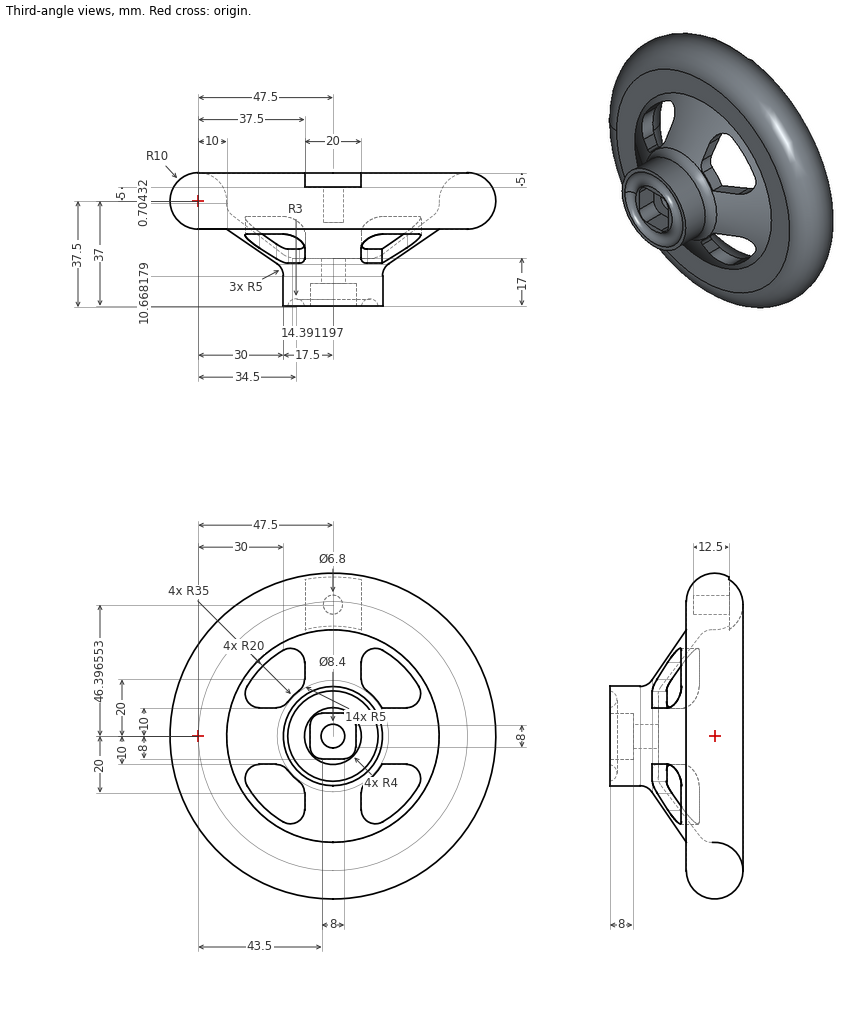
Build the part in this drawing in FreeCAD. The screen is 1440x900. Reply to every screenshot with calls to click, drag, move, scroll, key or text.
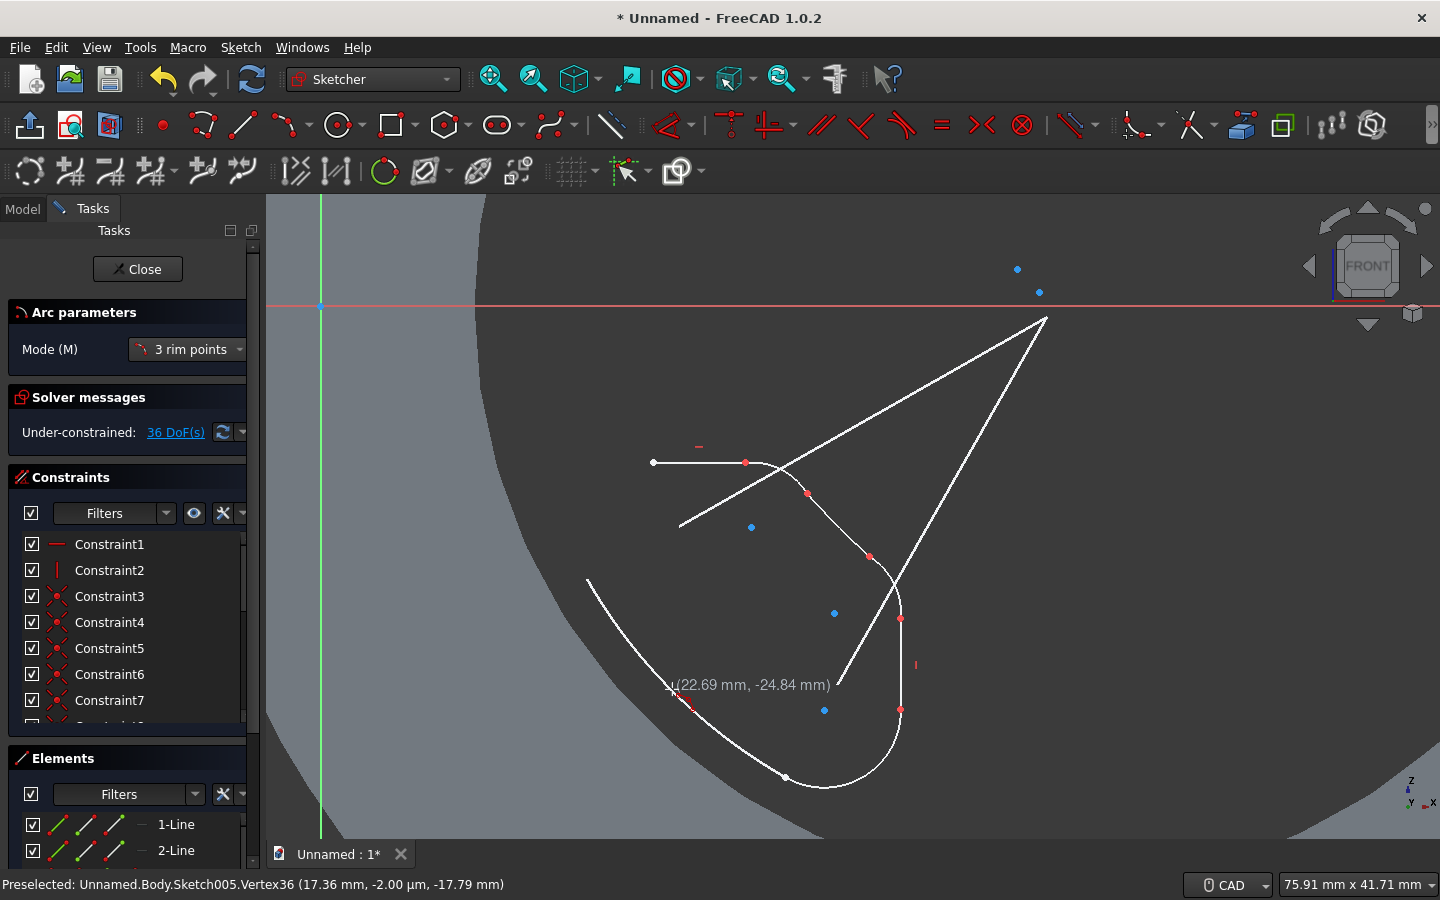
click(673, 689)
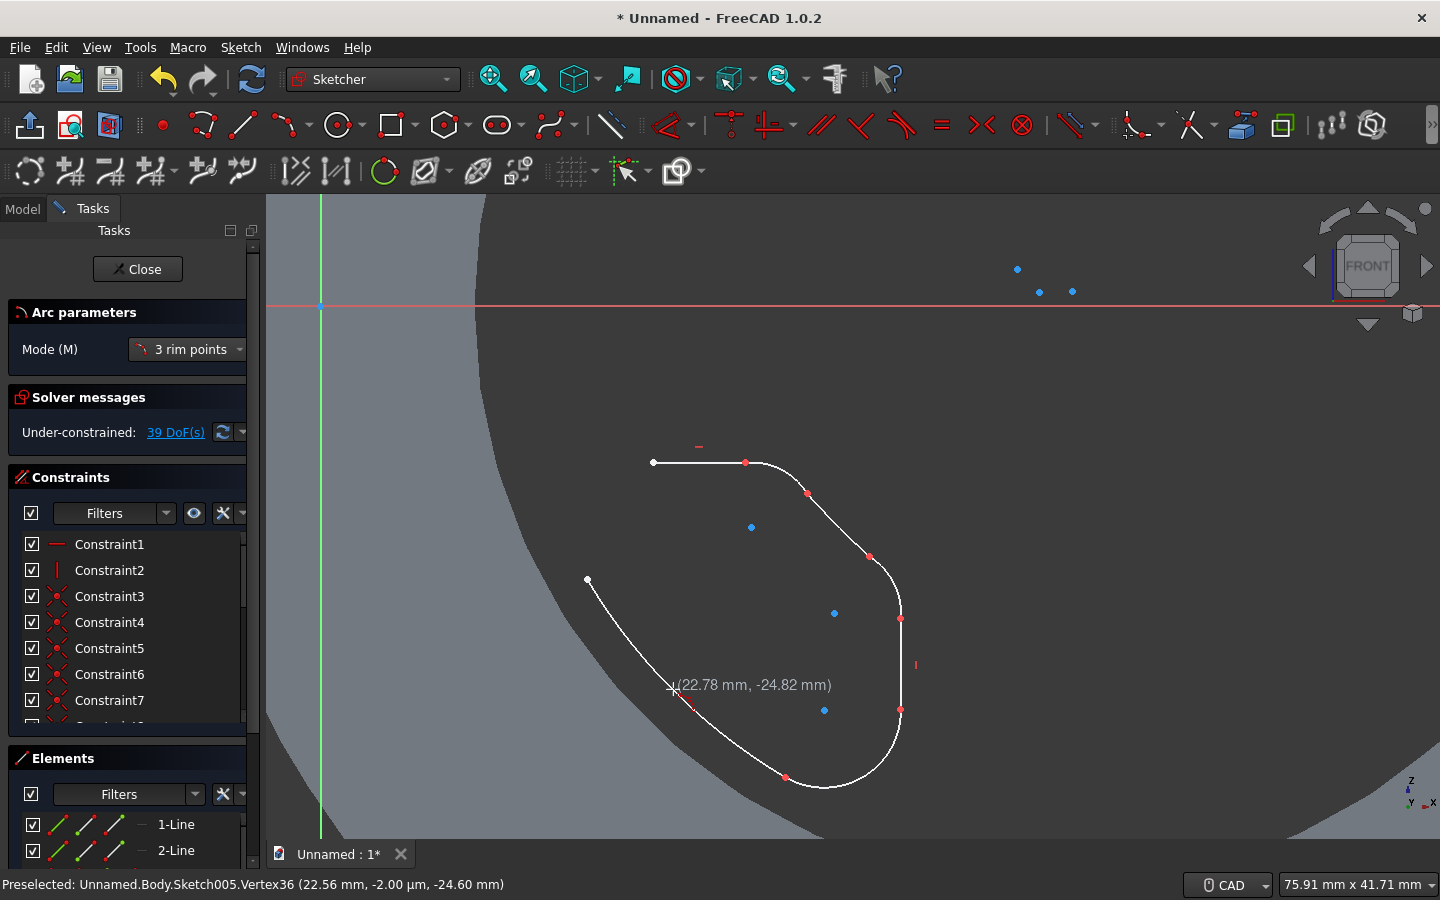
click(587, 579)
click(654, 463)
click(587, 499)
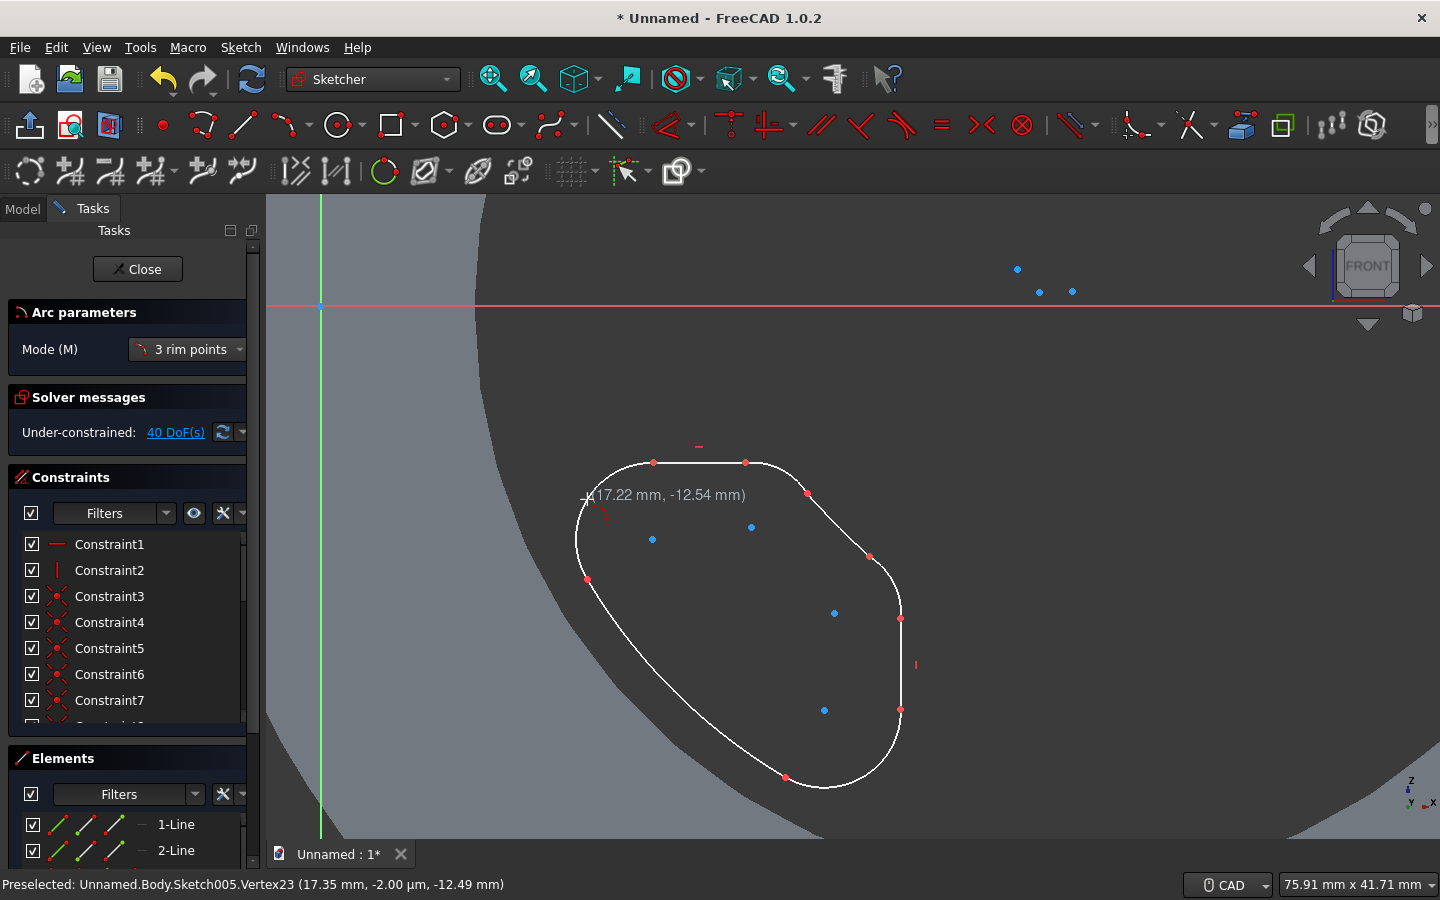
click(244, 126)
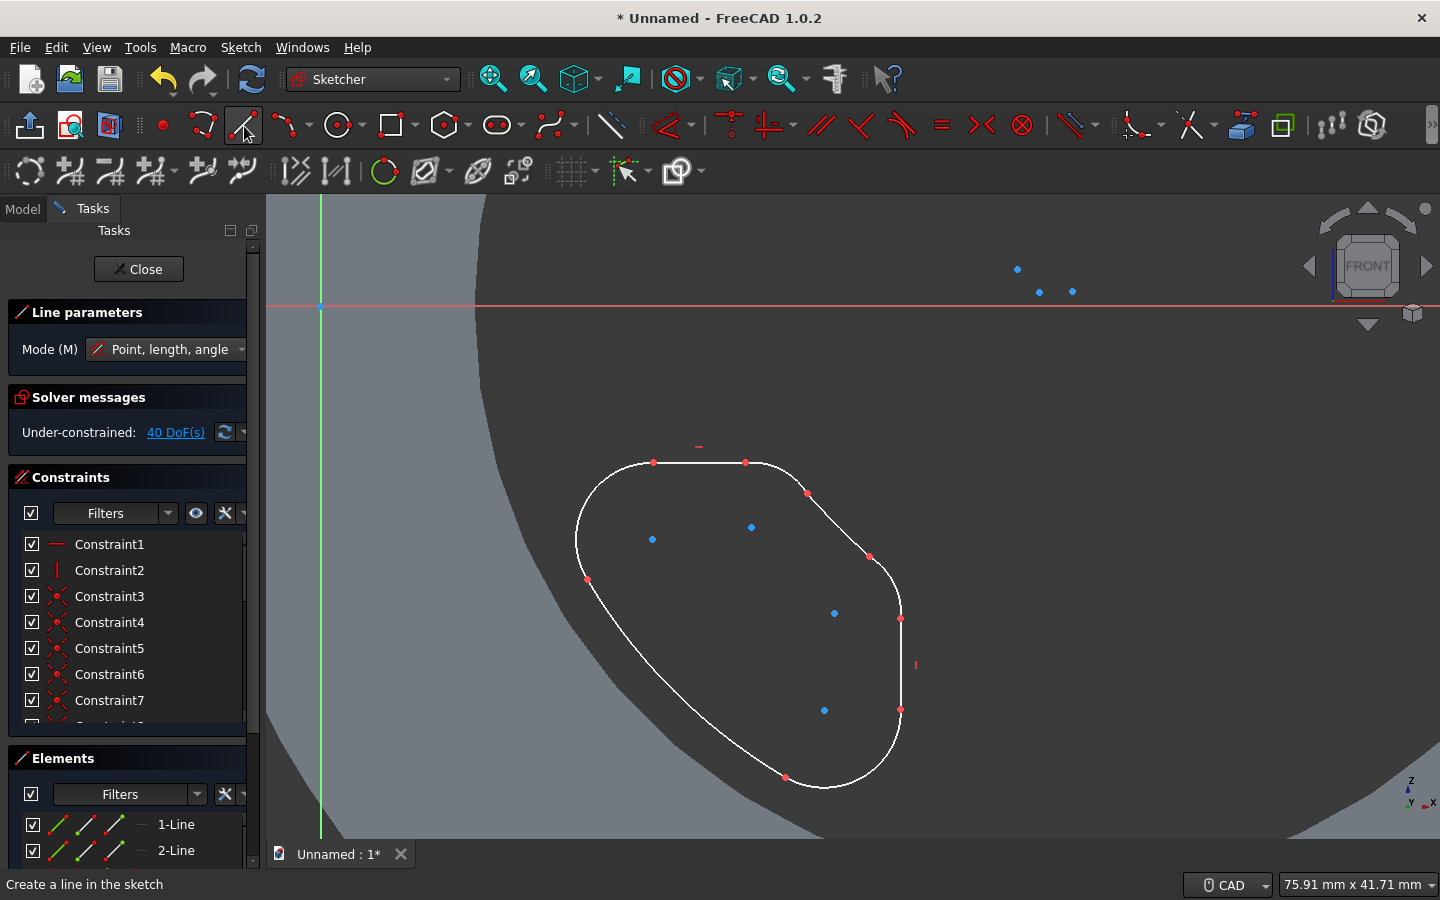
scroll(672, 688, down, 4)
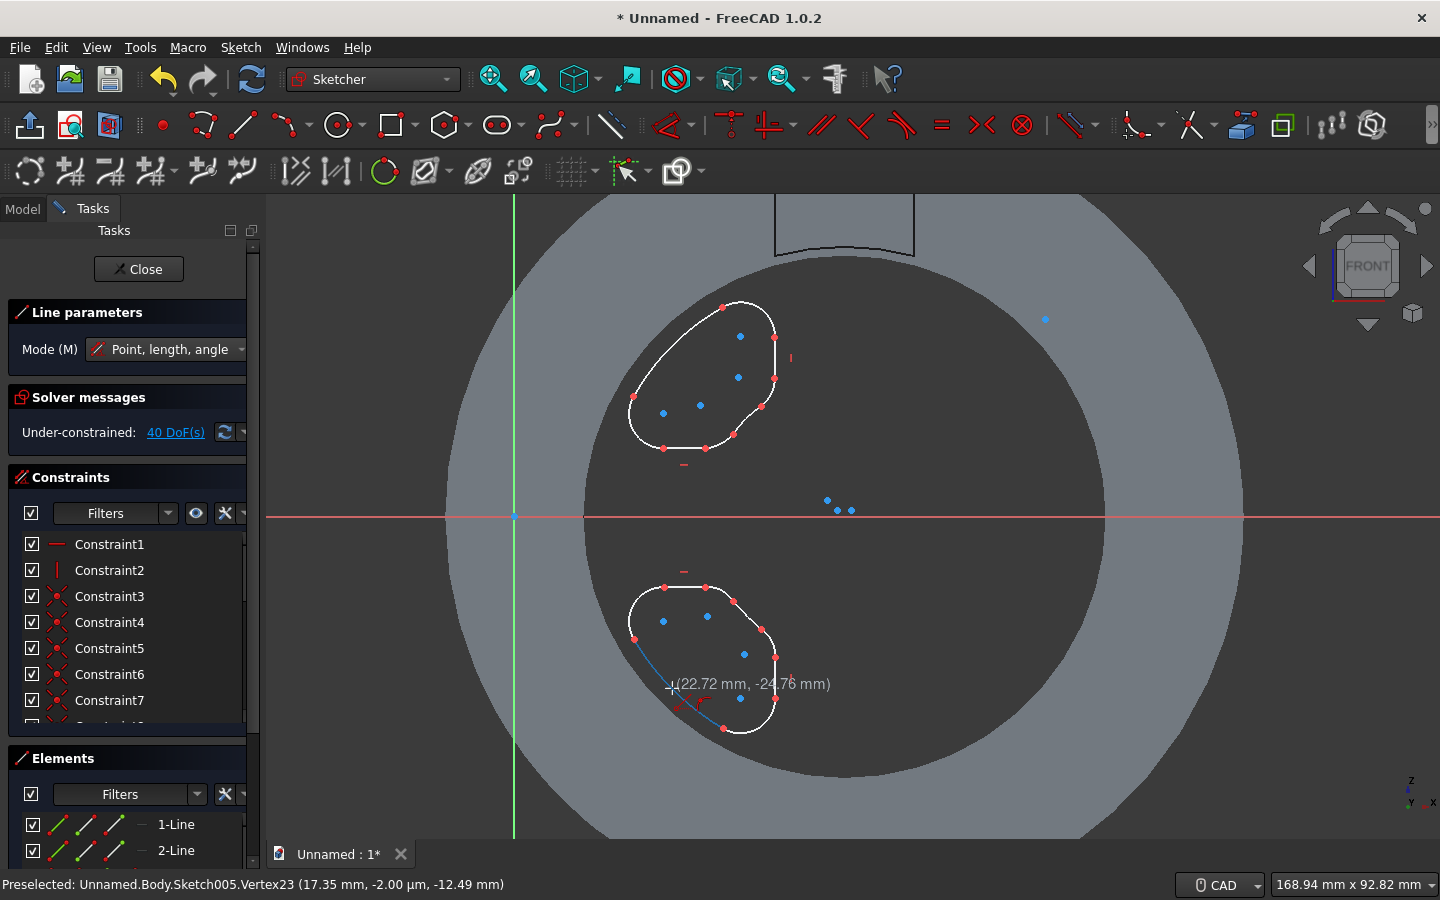
click(965, 586)
click(1025, 586)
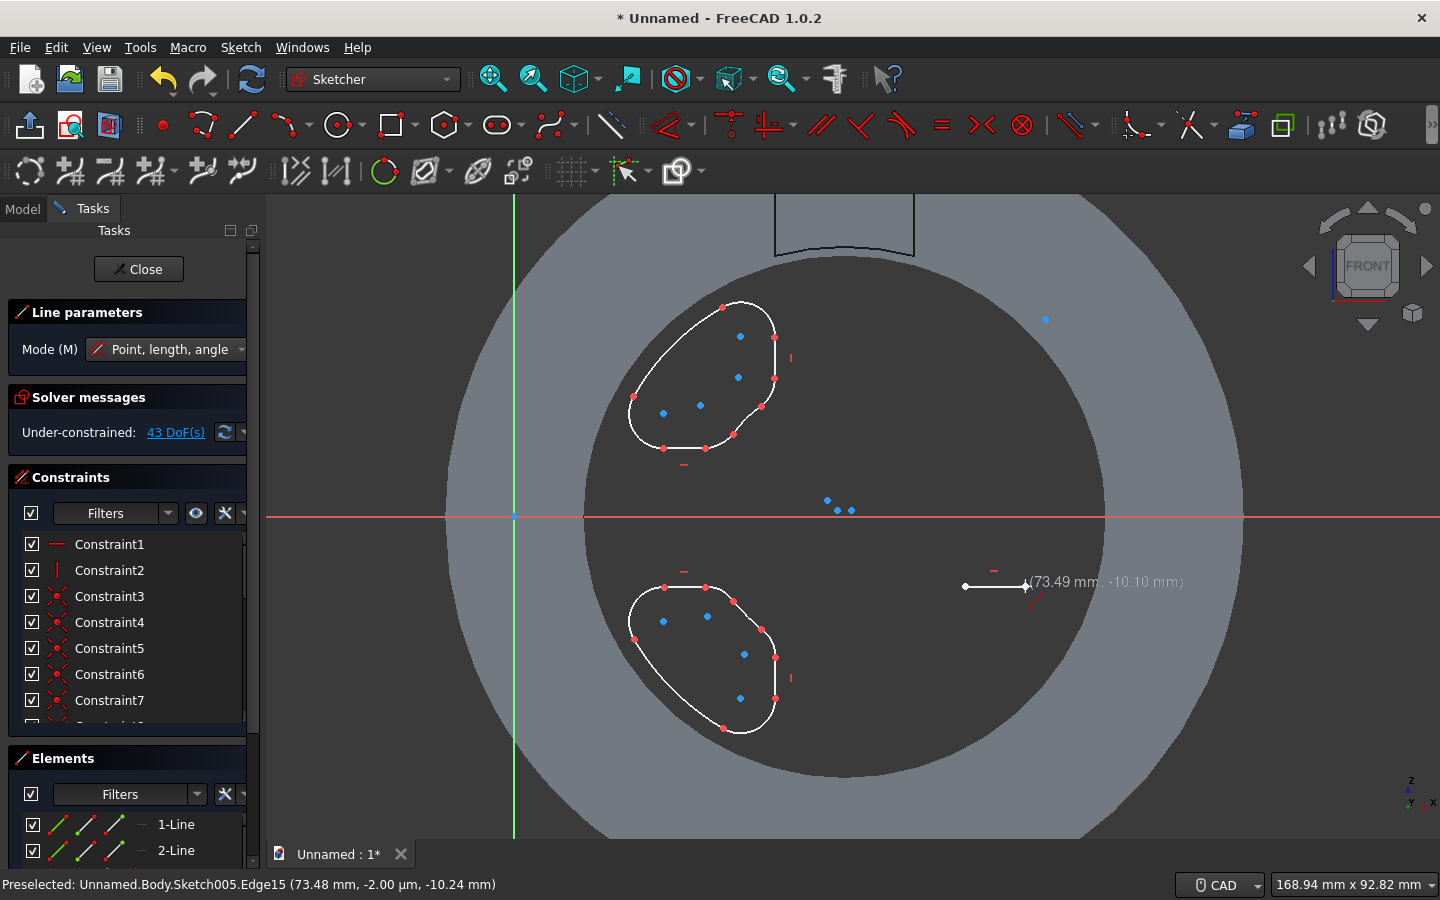
click(914, 697)
click(914, 656)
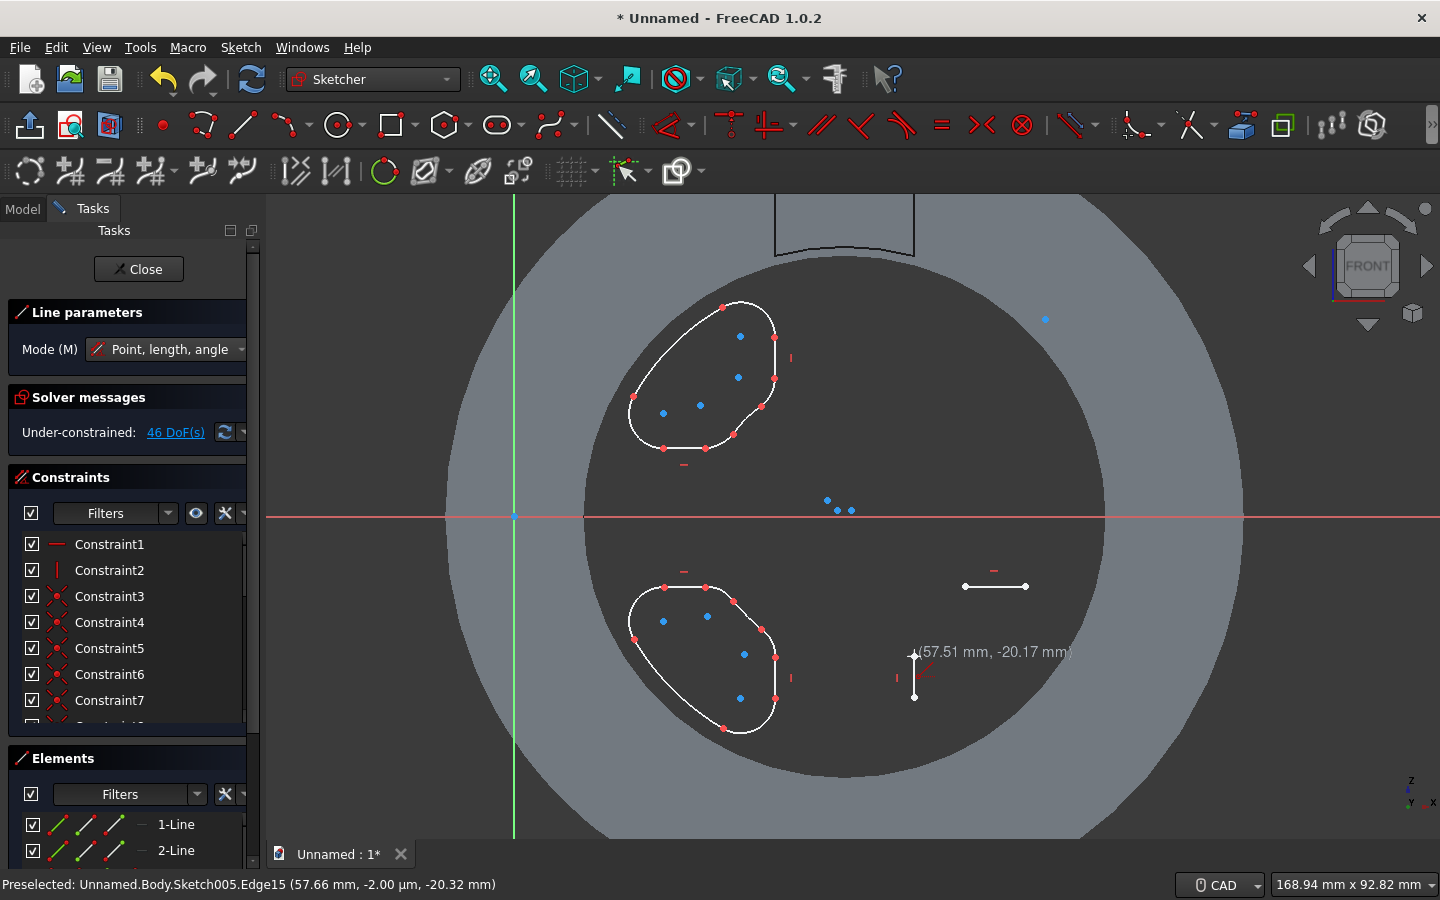
click(284, 126)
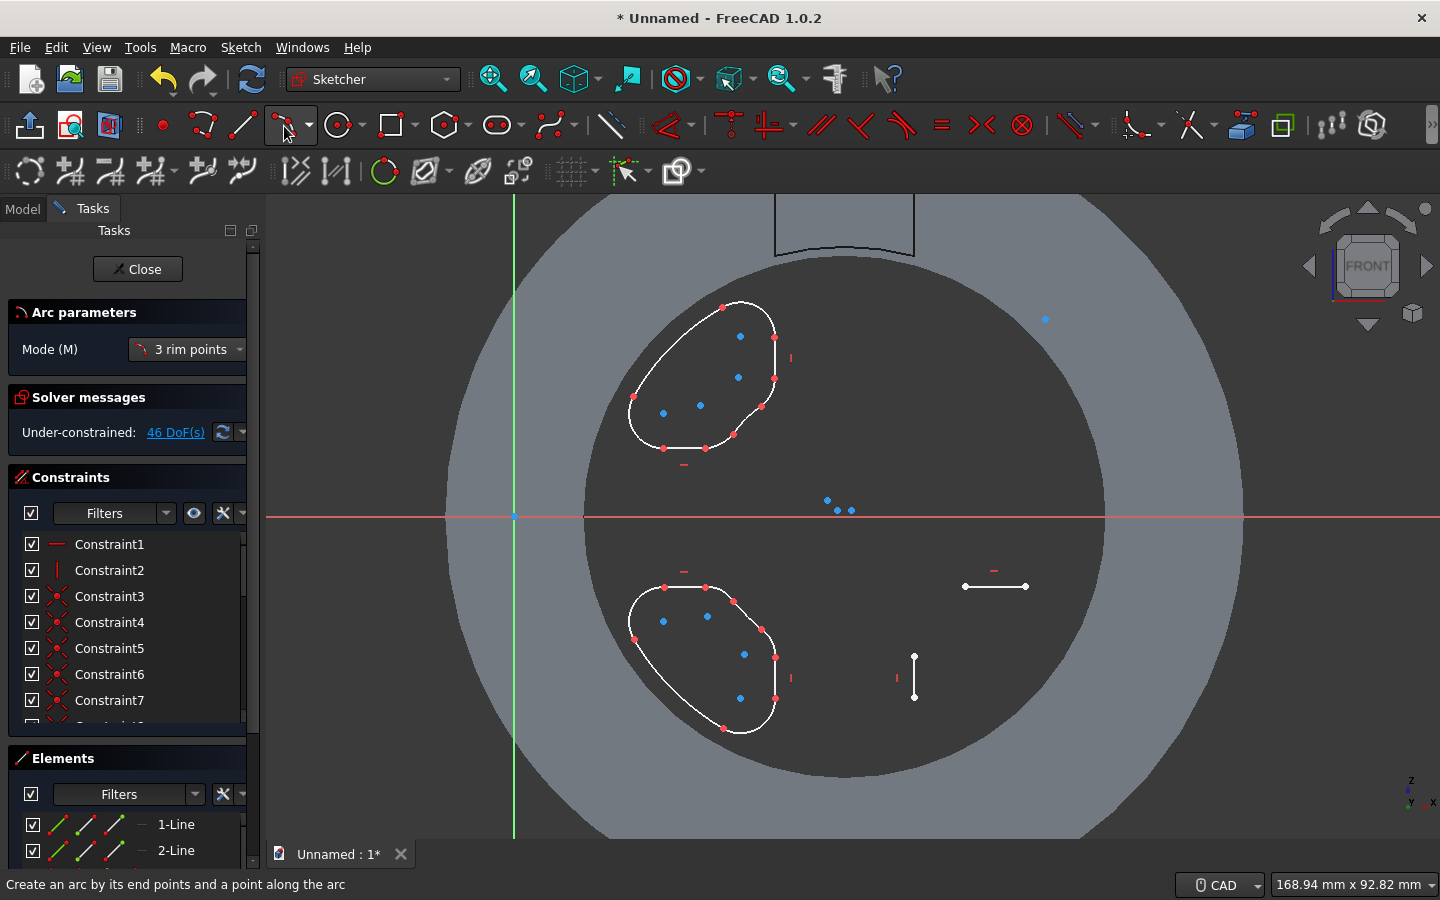
click(1025, 587)
click(1055, 638)
click(1055, 604)